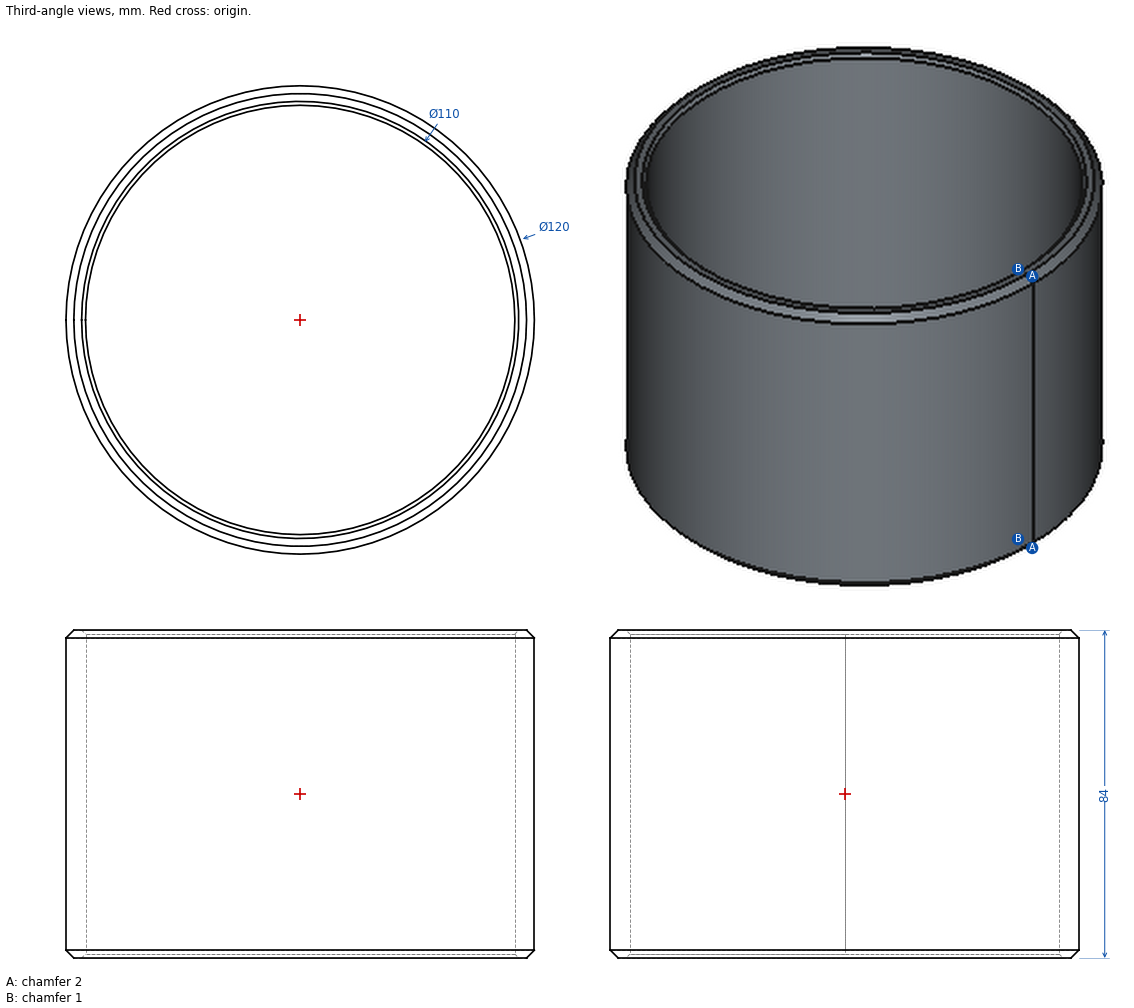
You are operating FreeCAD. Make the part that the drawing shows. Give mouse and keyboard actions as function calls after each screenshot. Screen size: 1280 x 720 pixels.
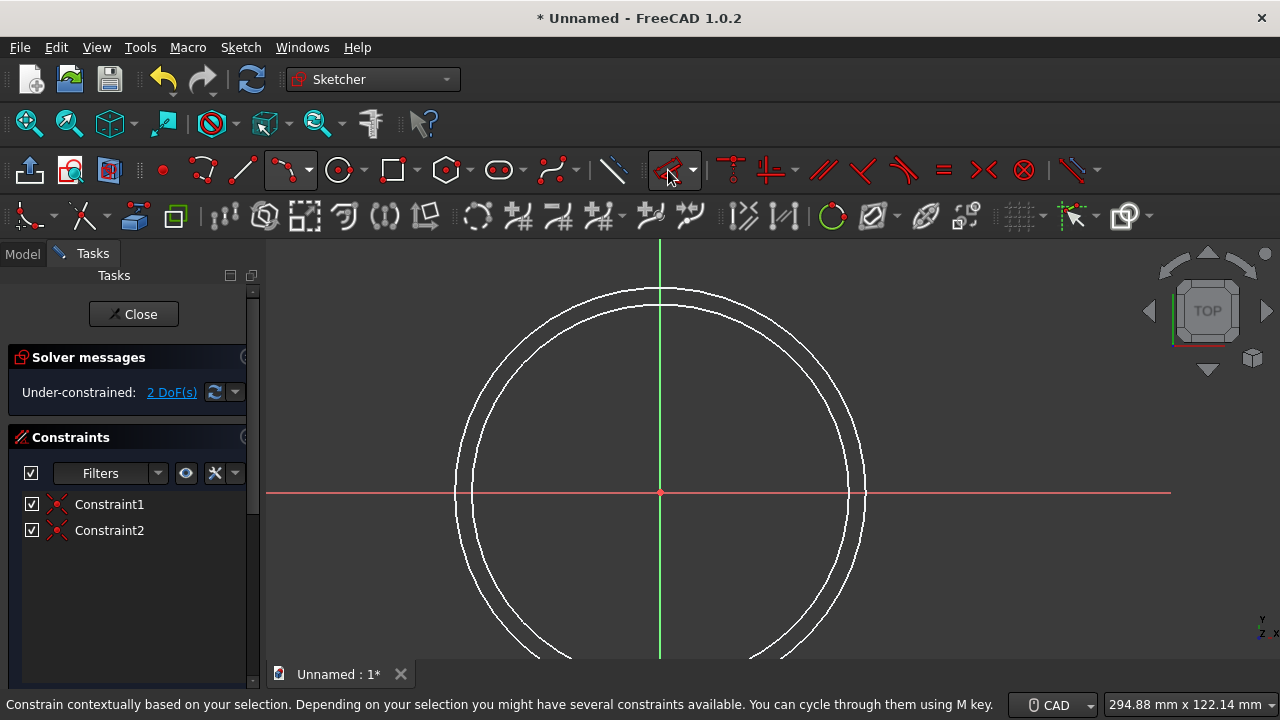
click(805, 347)
click(828, 324)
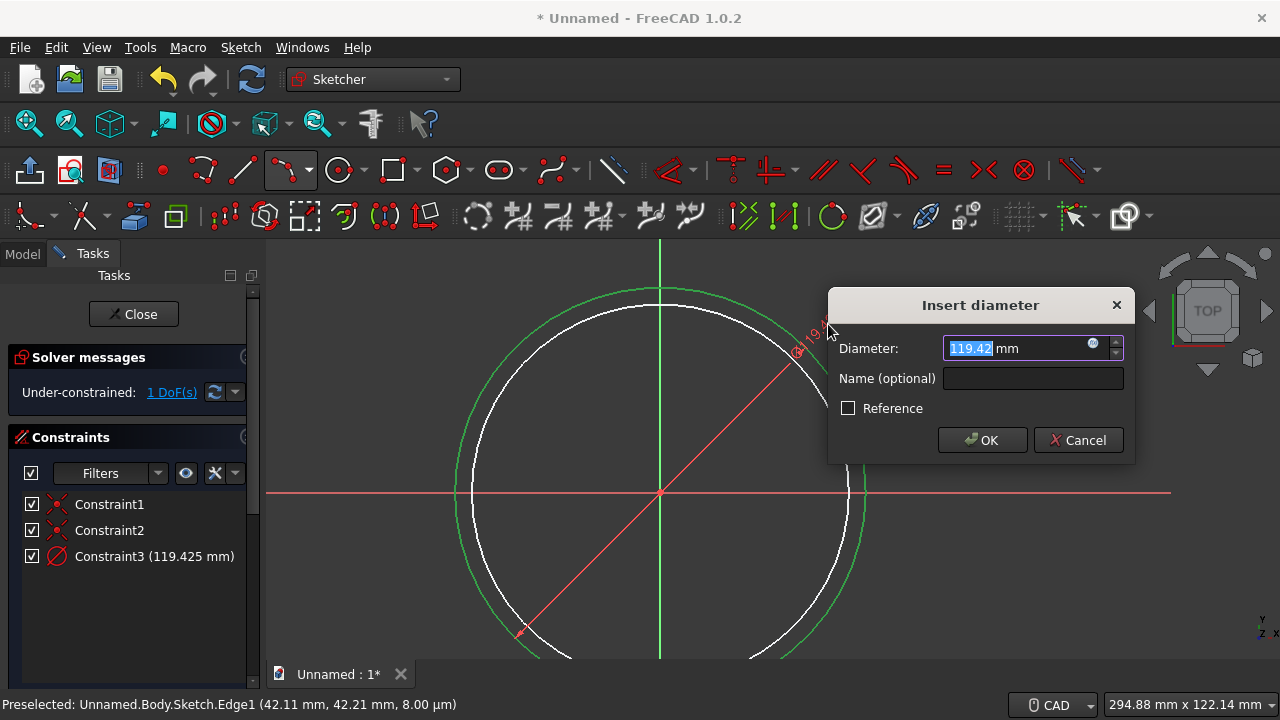
text(120)
key(Return)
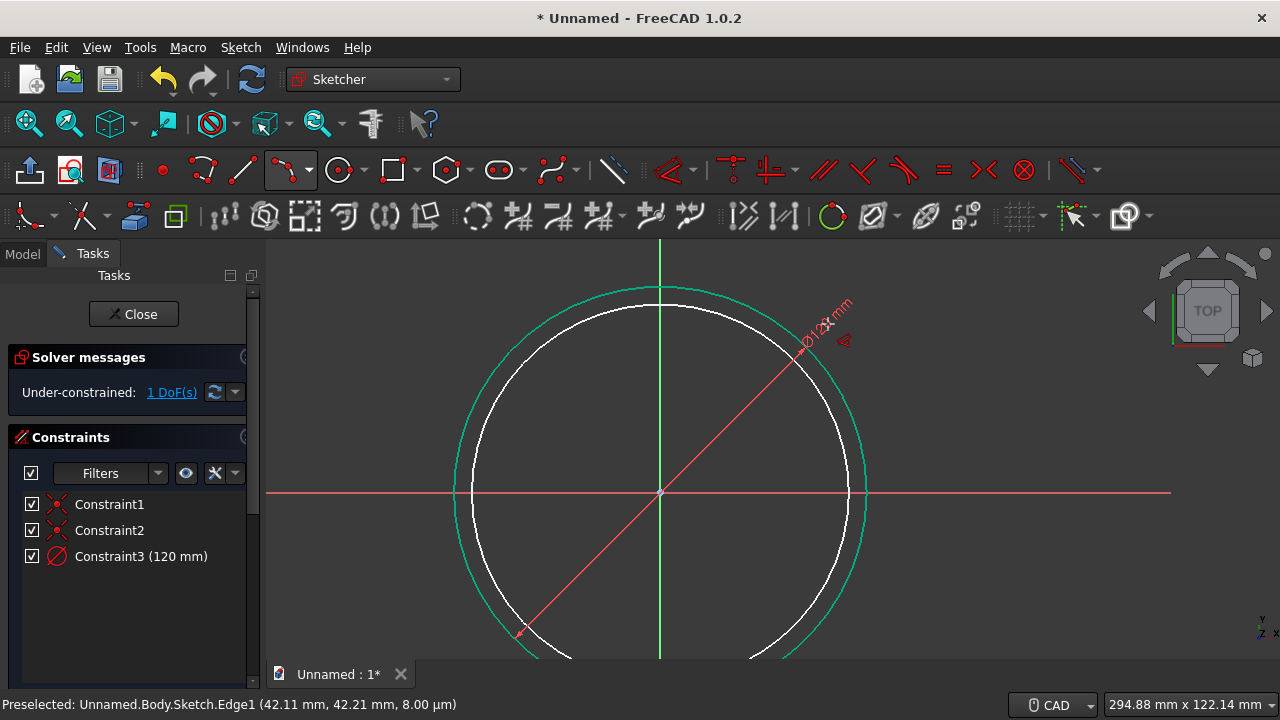
click(793, 359)
click(872, 430)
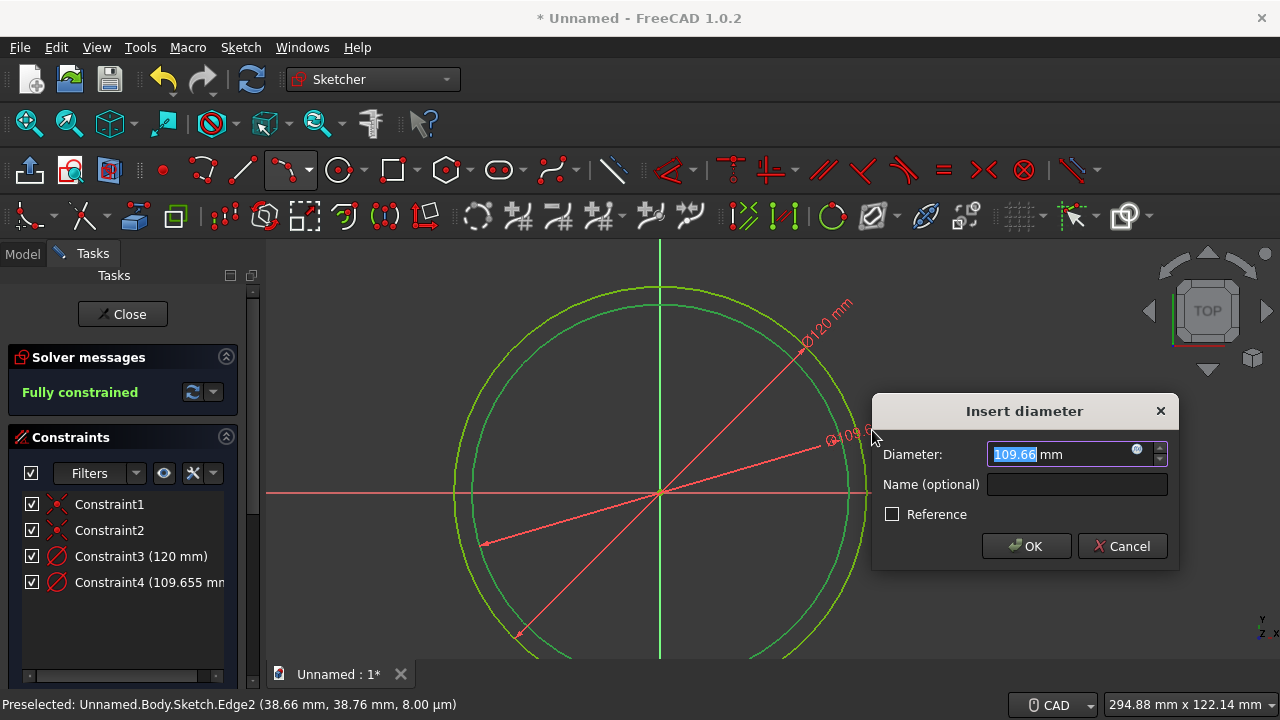
text(110)
key(Return)
key(Escape)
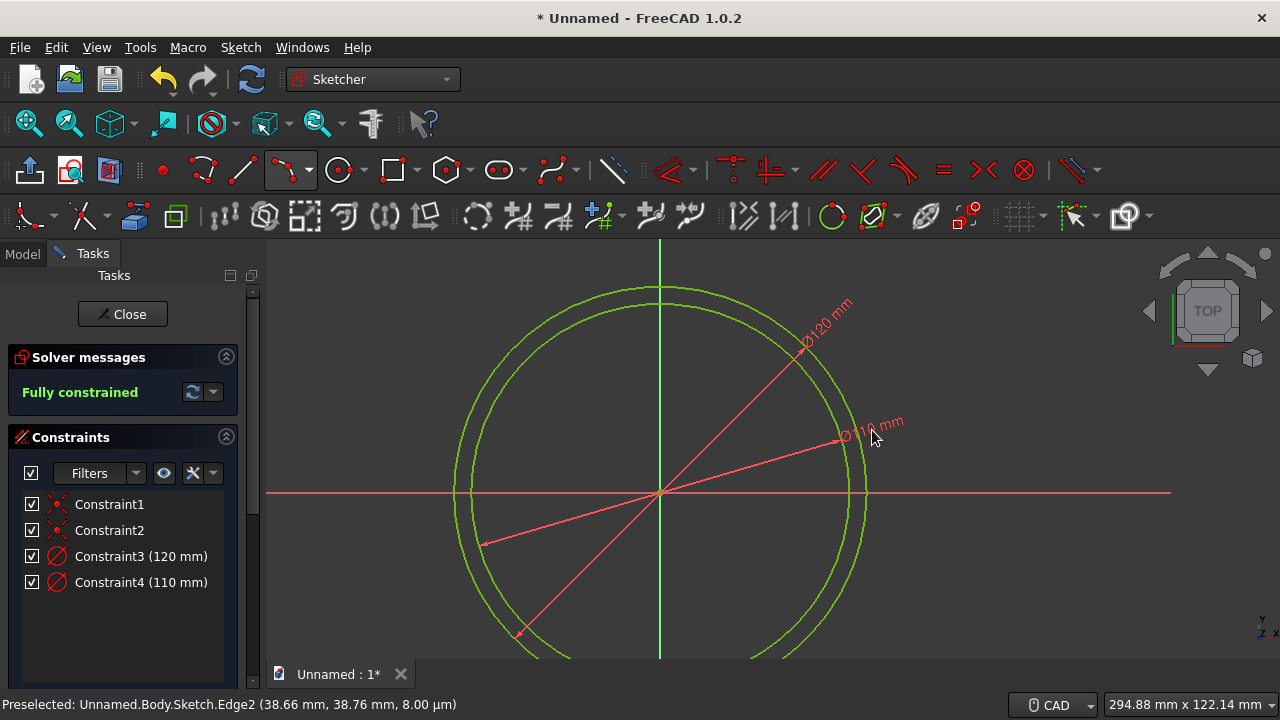
click(123, 314)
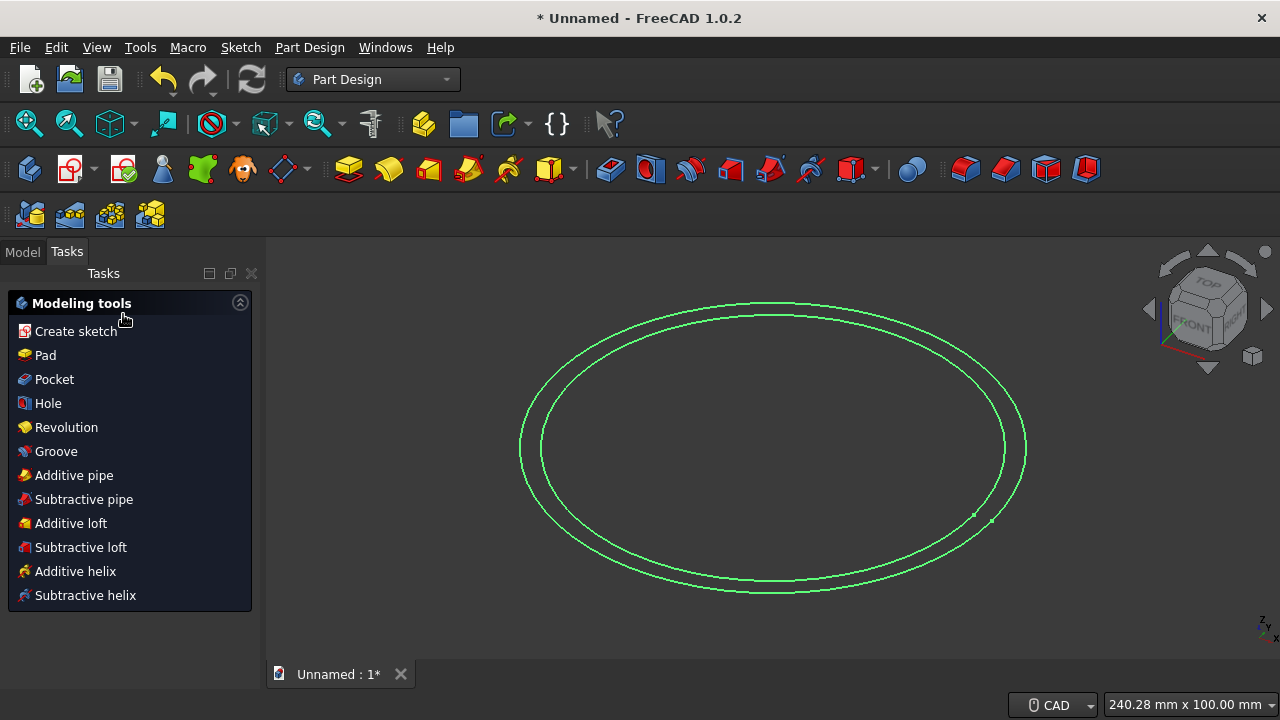
click(350, 170)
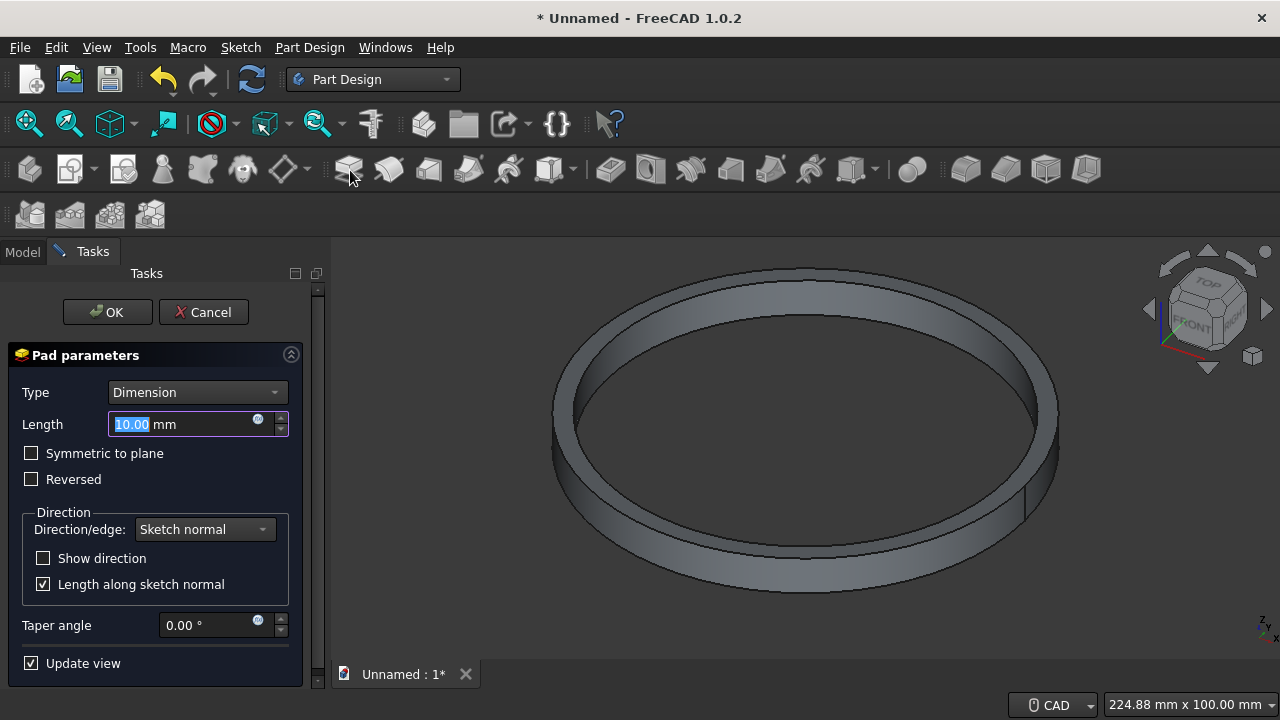
text(84)
key(Tab)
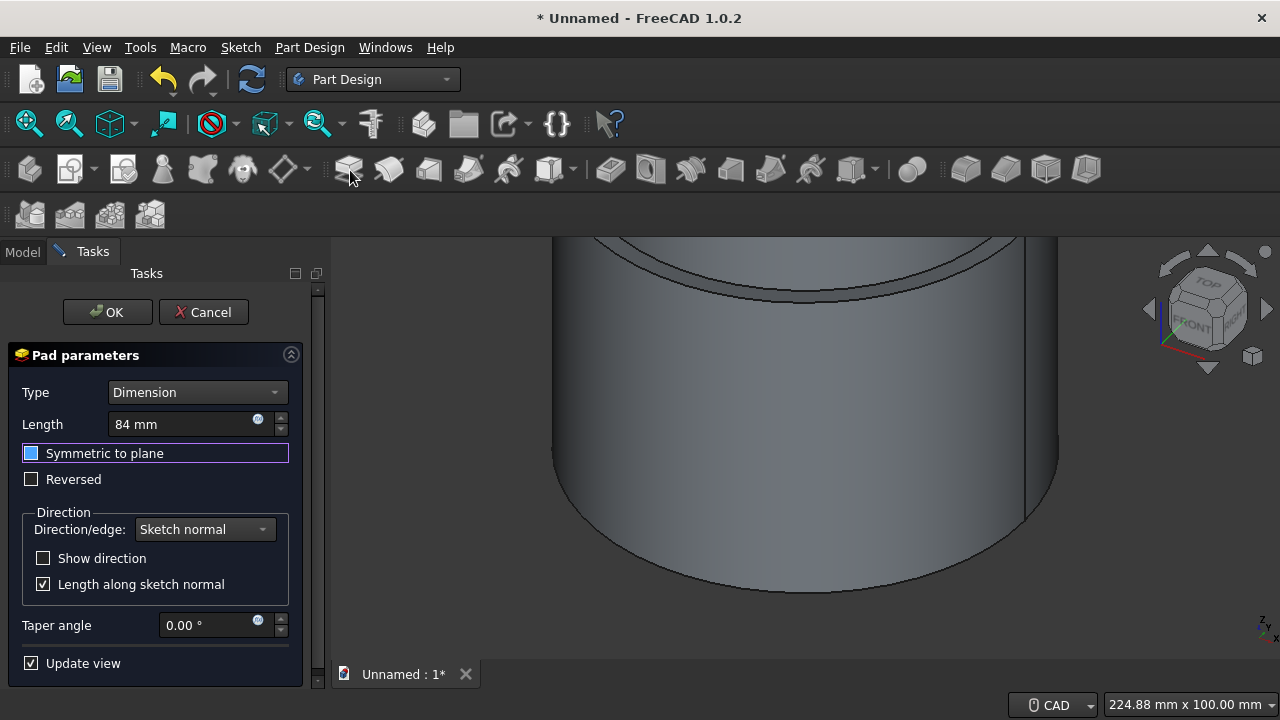
click(30, 453)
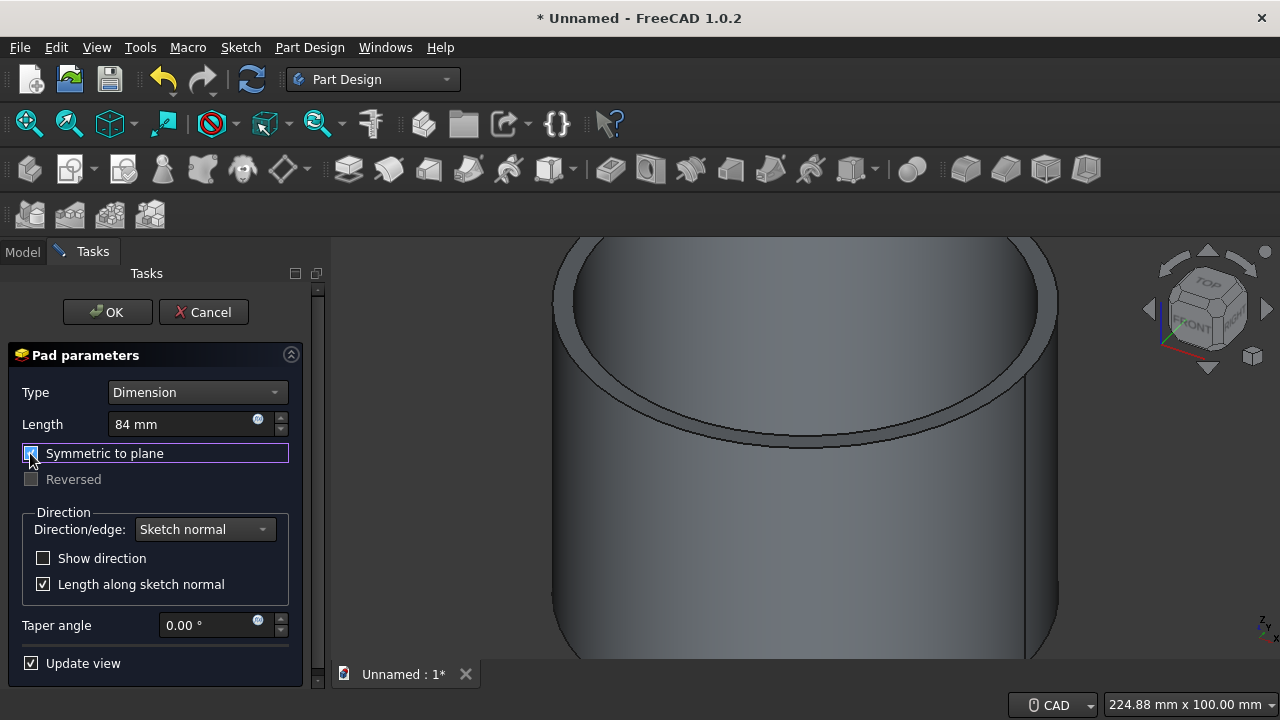
click(108, 312)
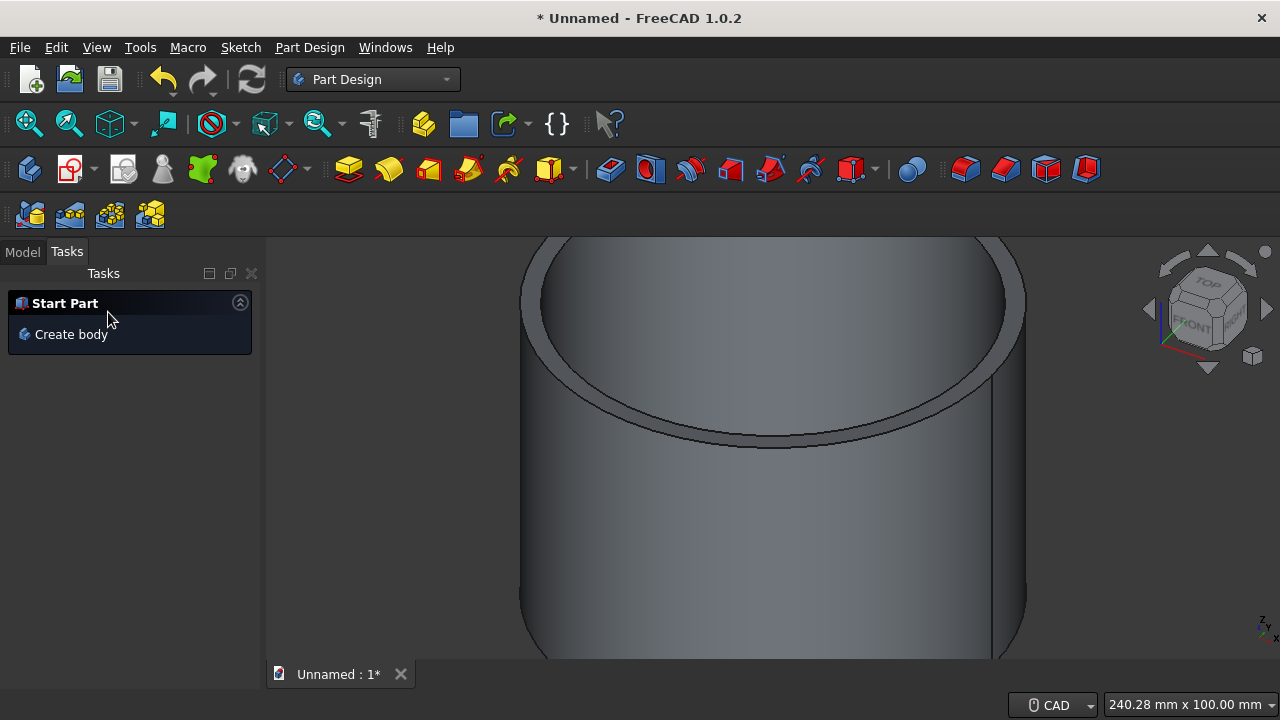
click(30, 124)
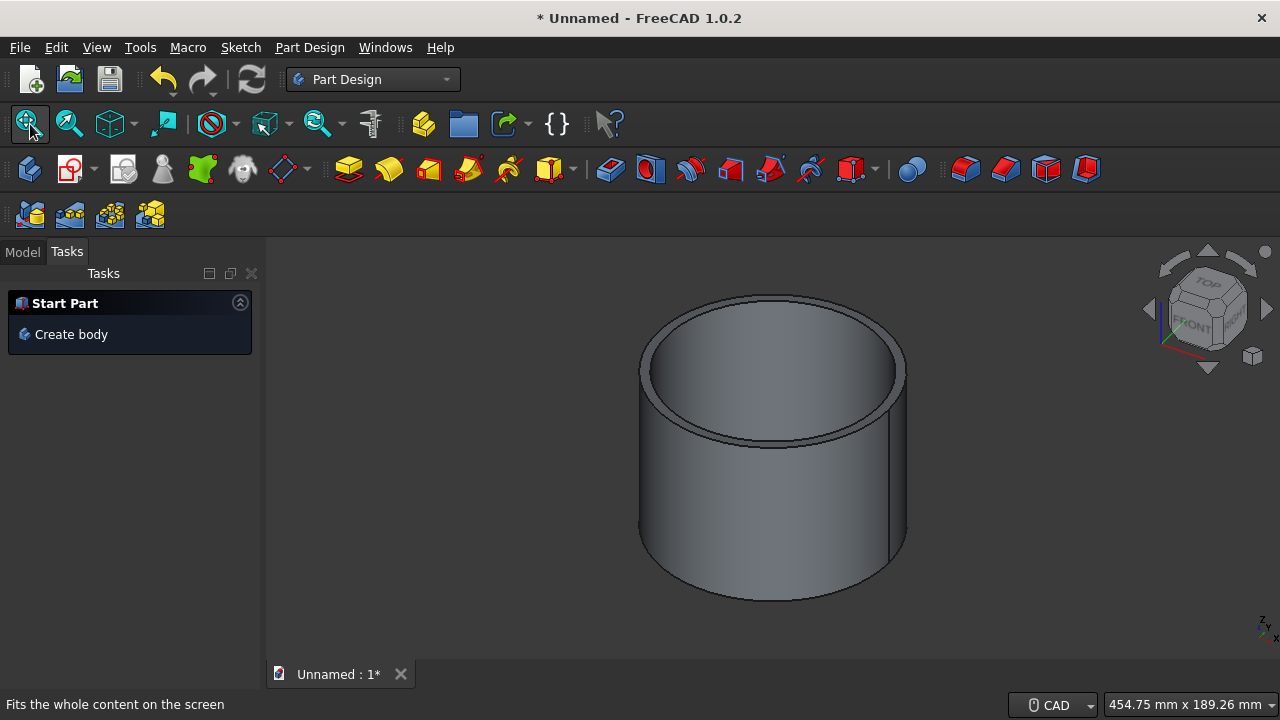
click(640, 378)